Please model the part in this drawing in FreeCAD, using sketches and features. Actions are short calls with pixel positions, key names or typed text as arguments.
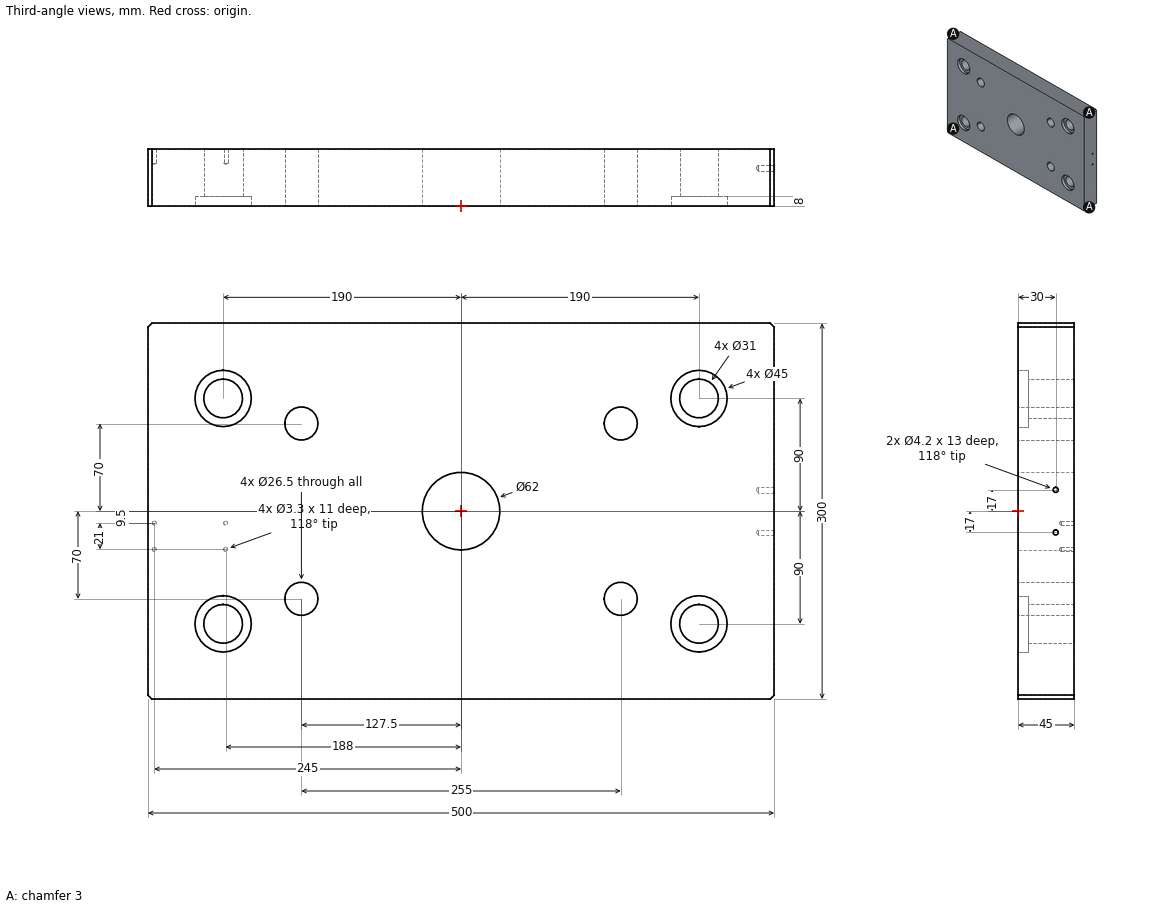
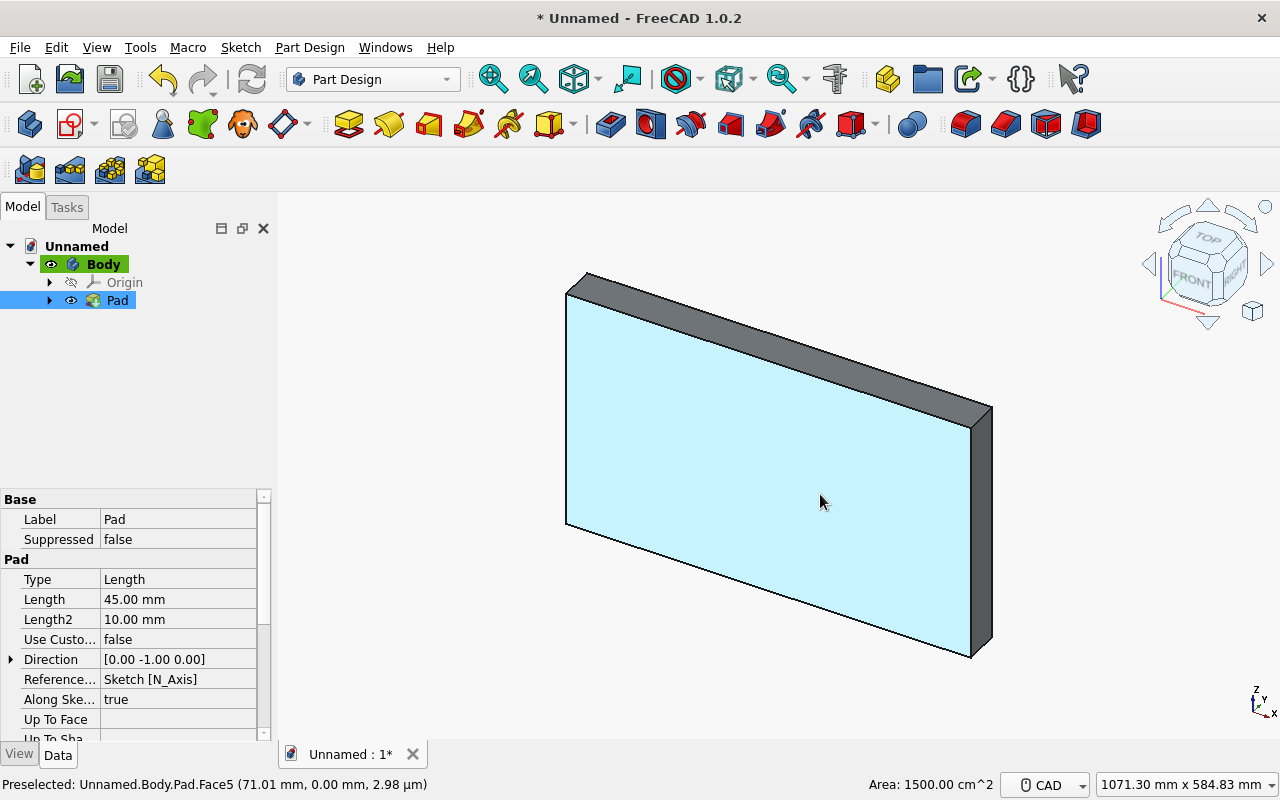
click(70, 124)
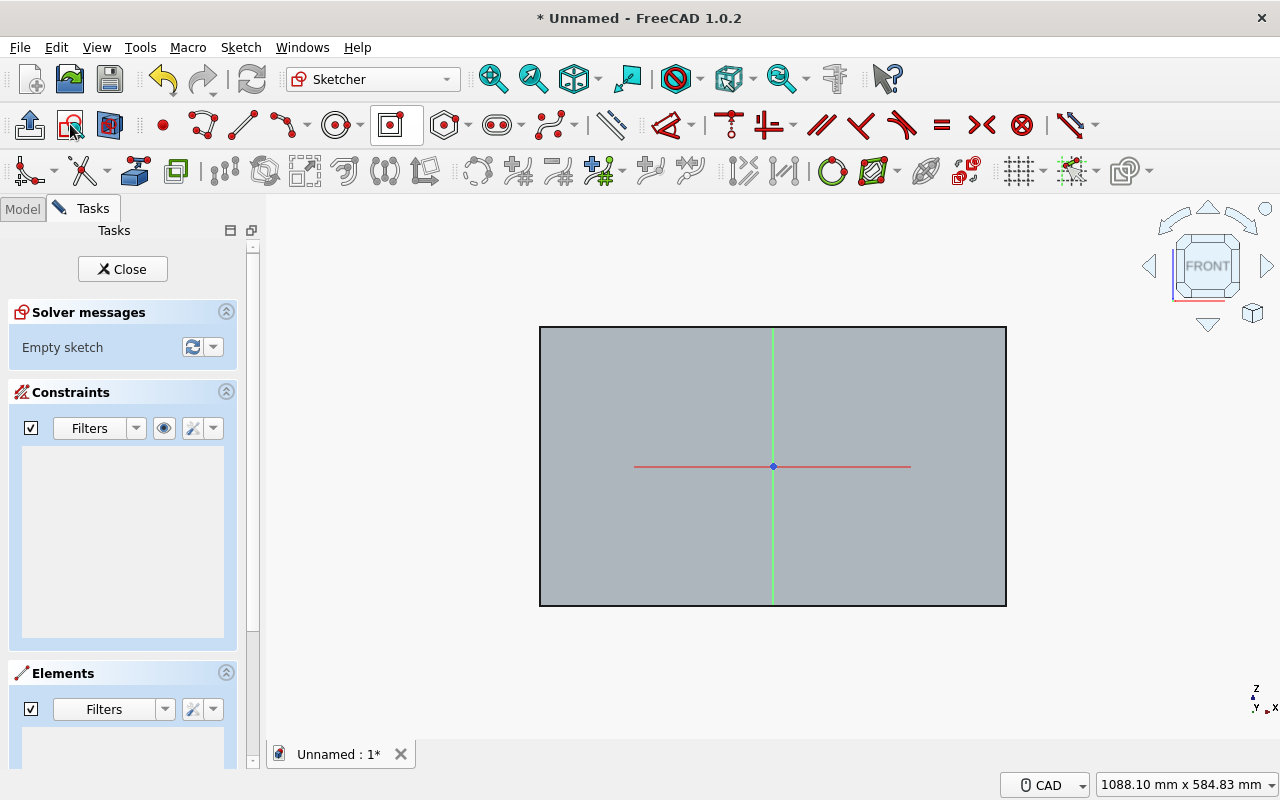
scroll(912, 467, up, 2)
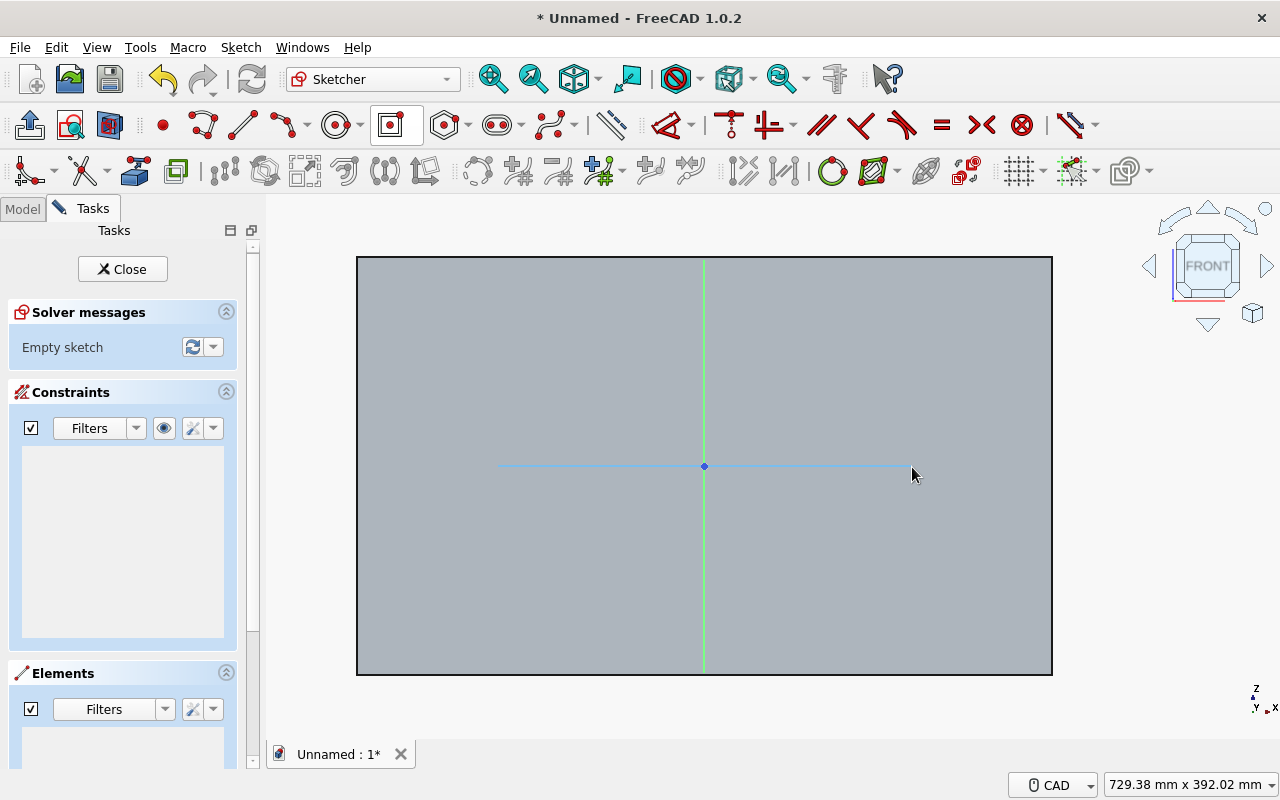
key(g)
key(c)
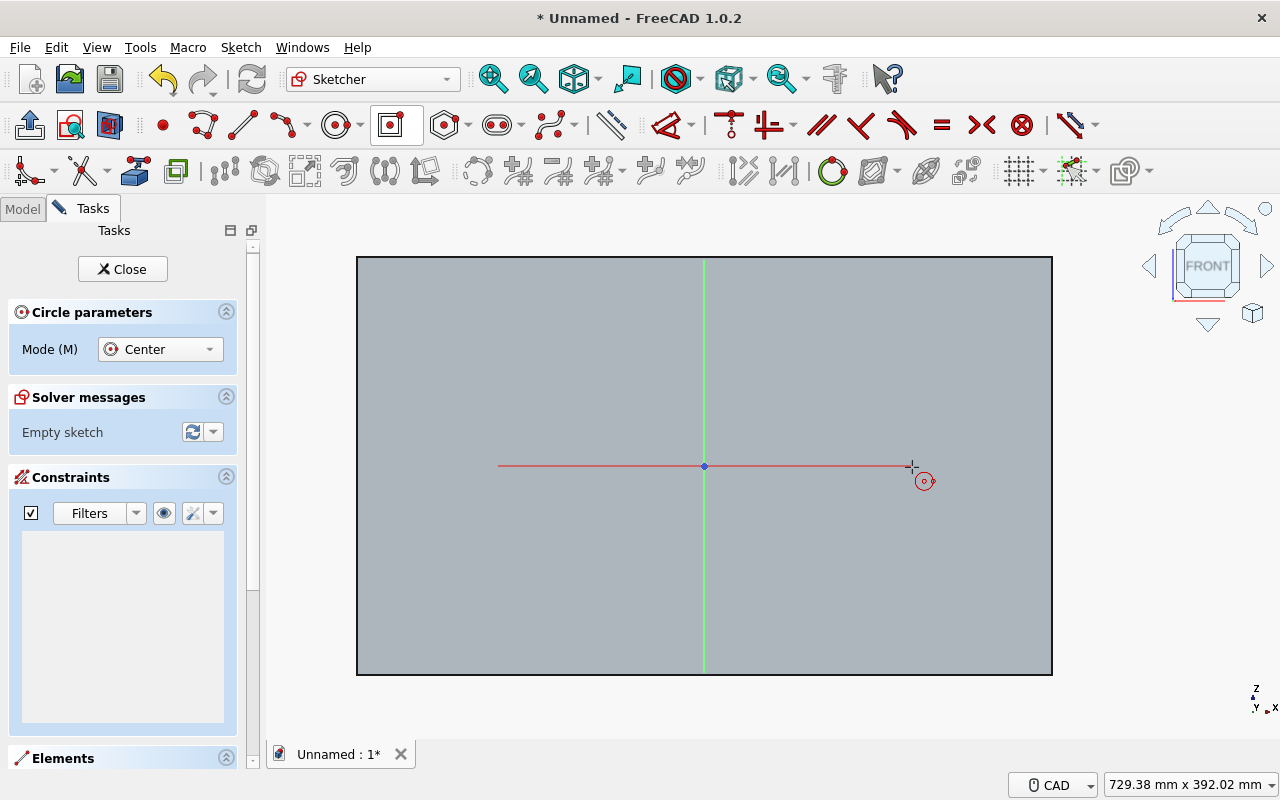
click(968, 341)
click(991, 319)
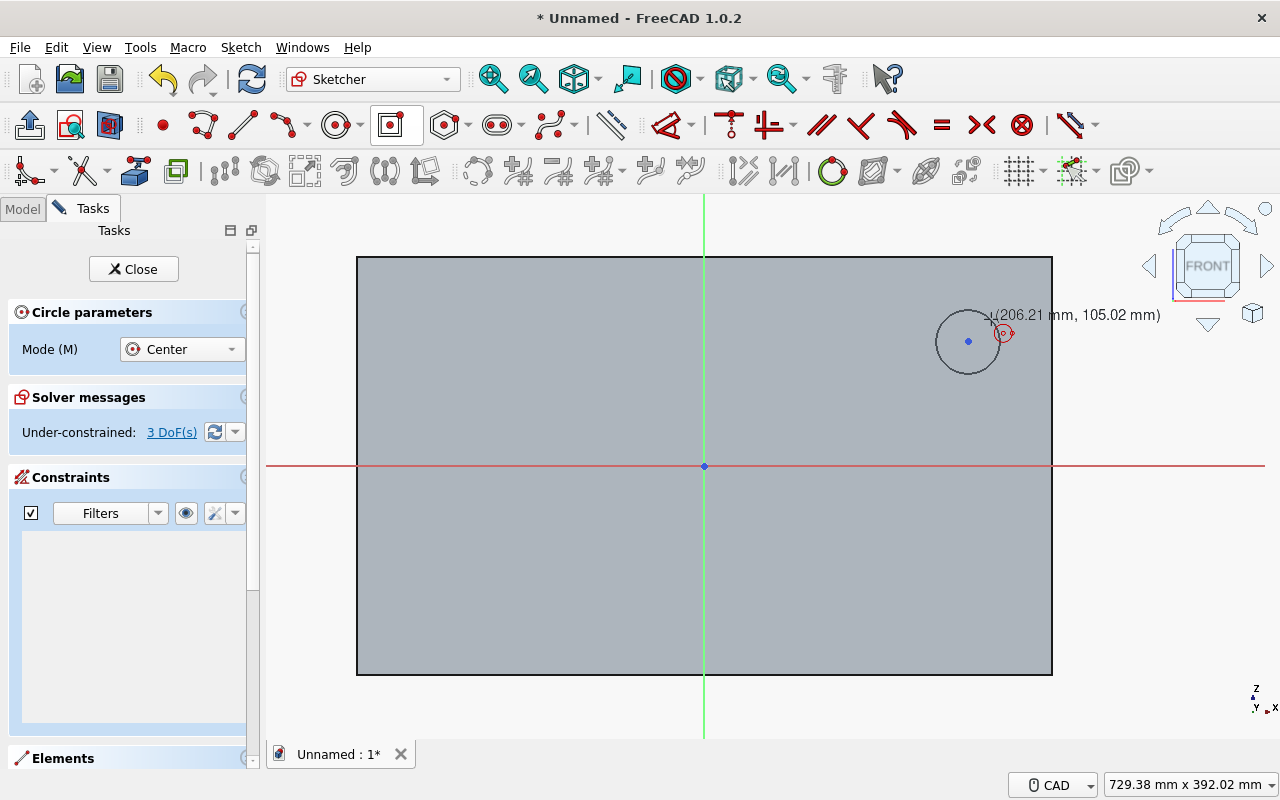
click(440, 341)
click(462, 319)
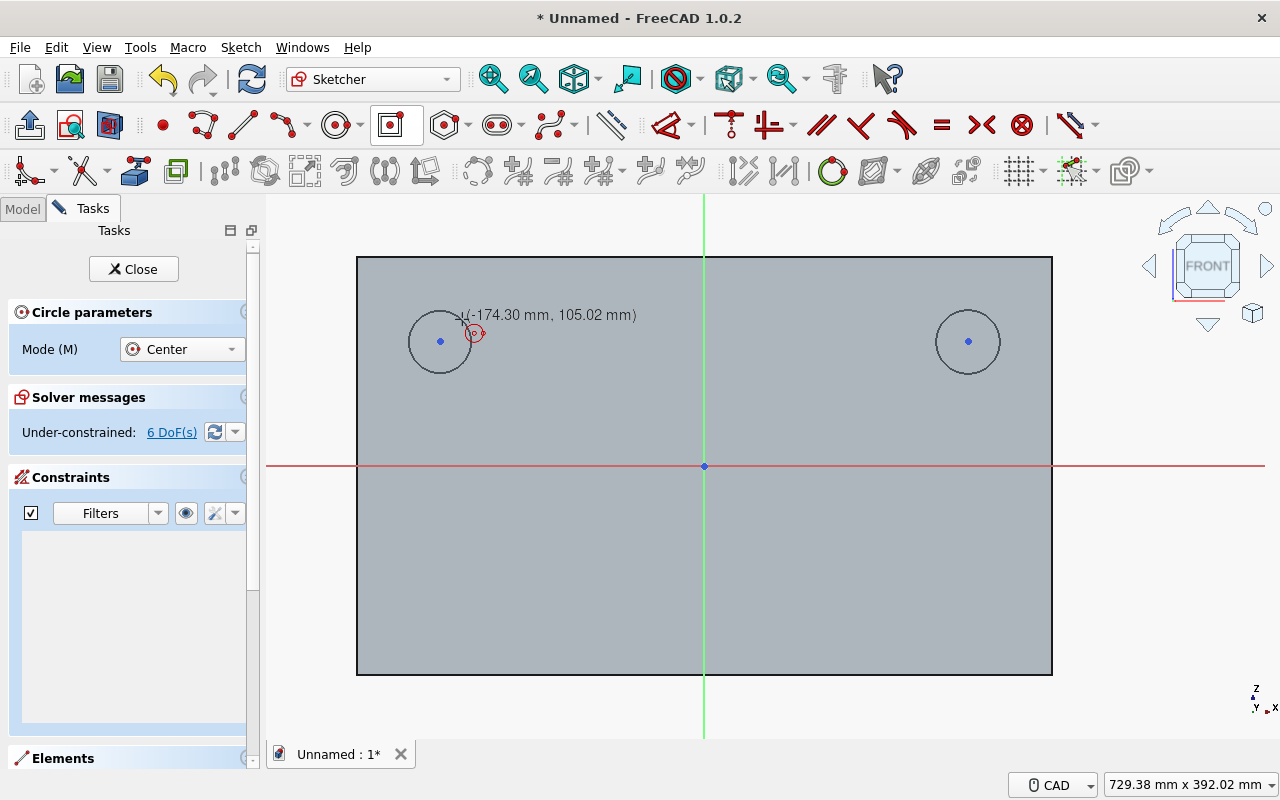
click(968, 591)
click(991, 569)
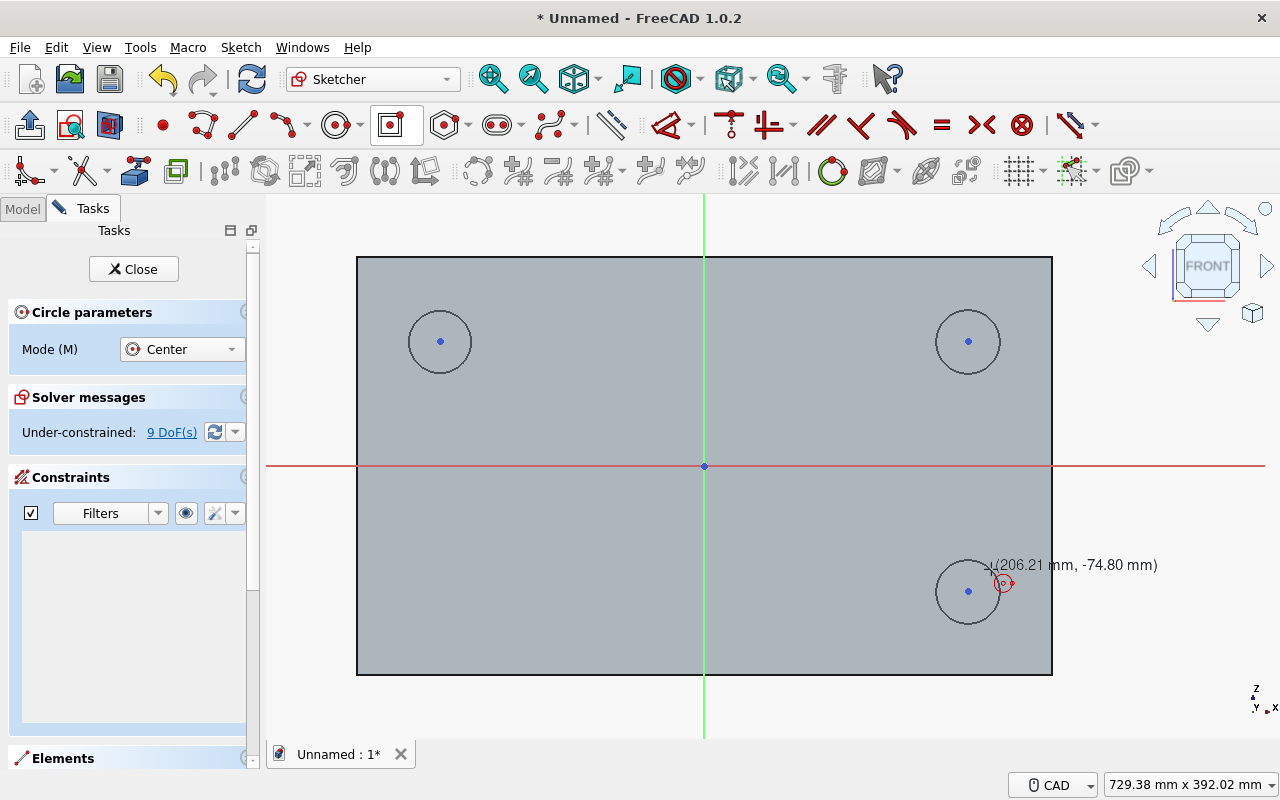
click(440, 591)
click(462, 569)
key(Escape)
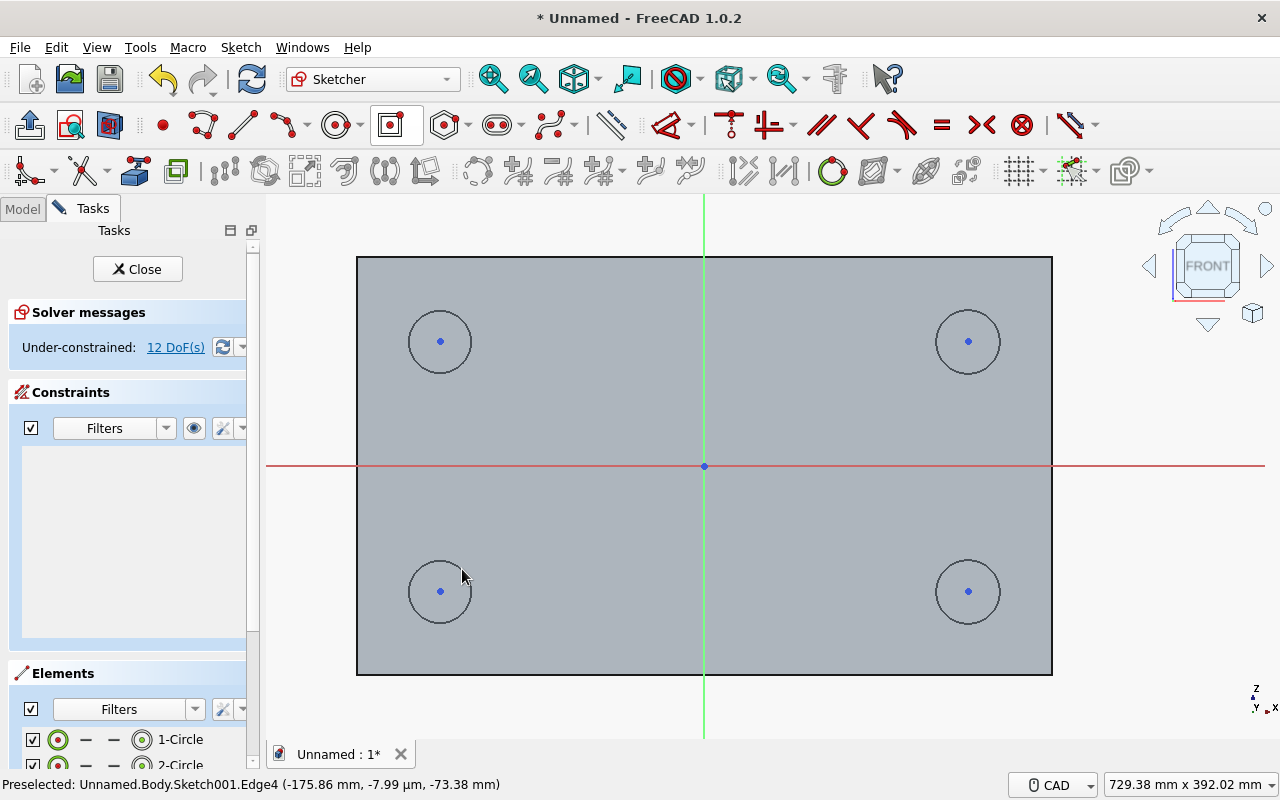
click(990, 319)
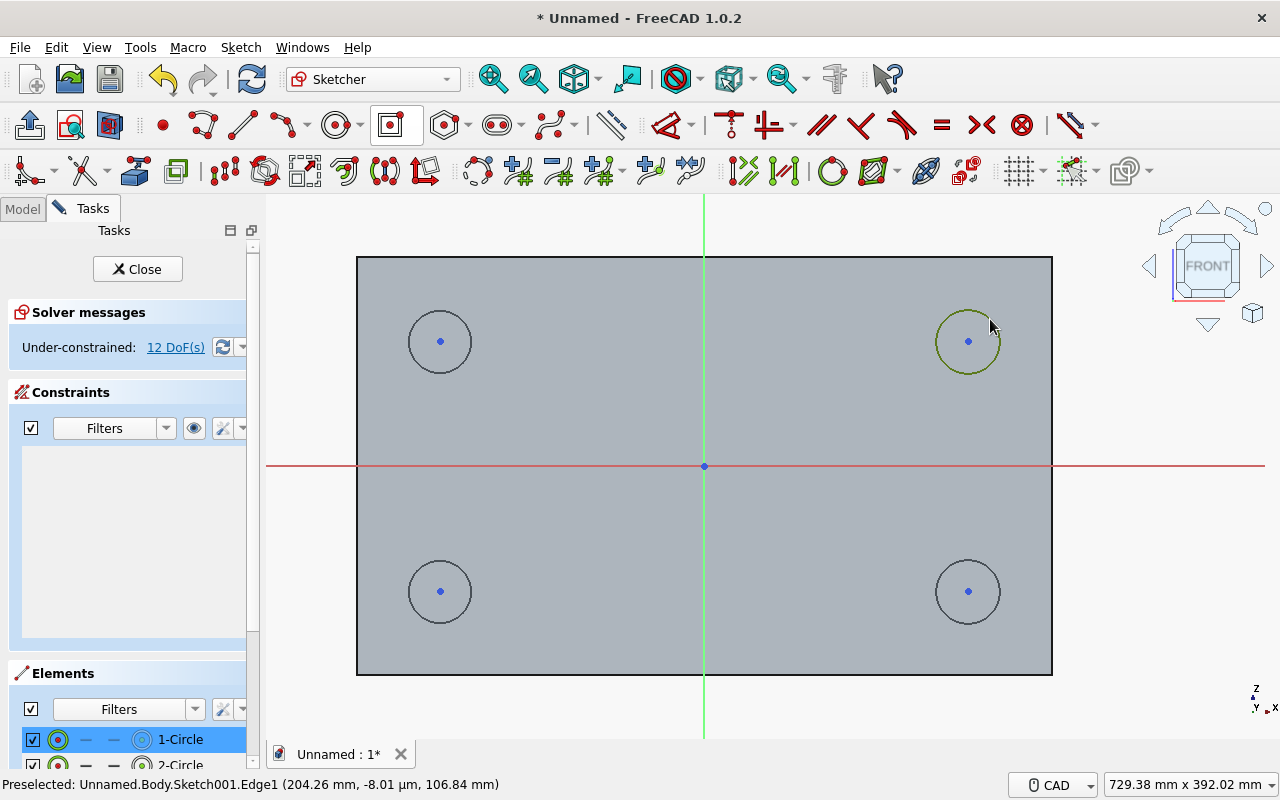
click(462, 320)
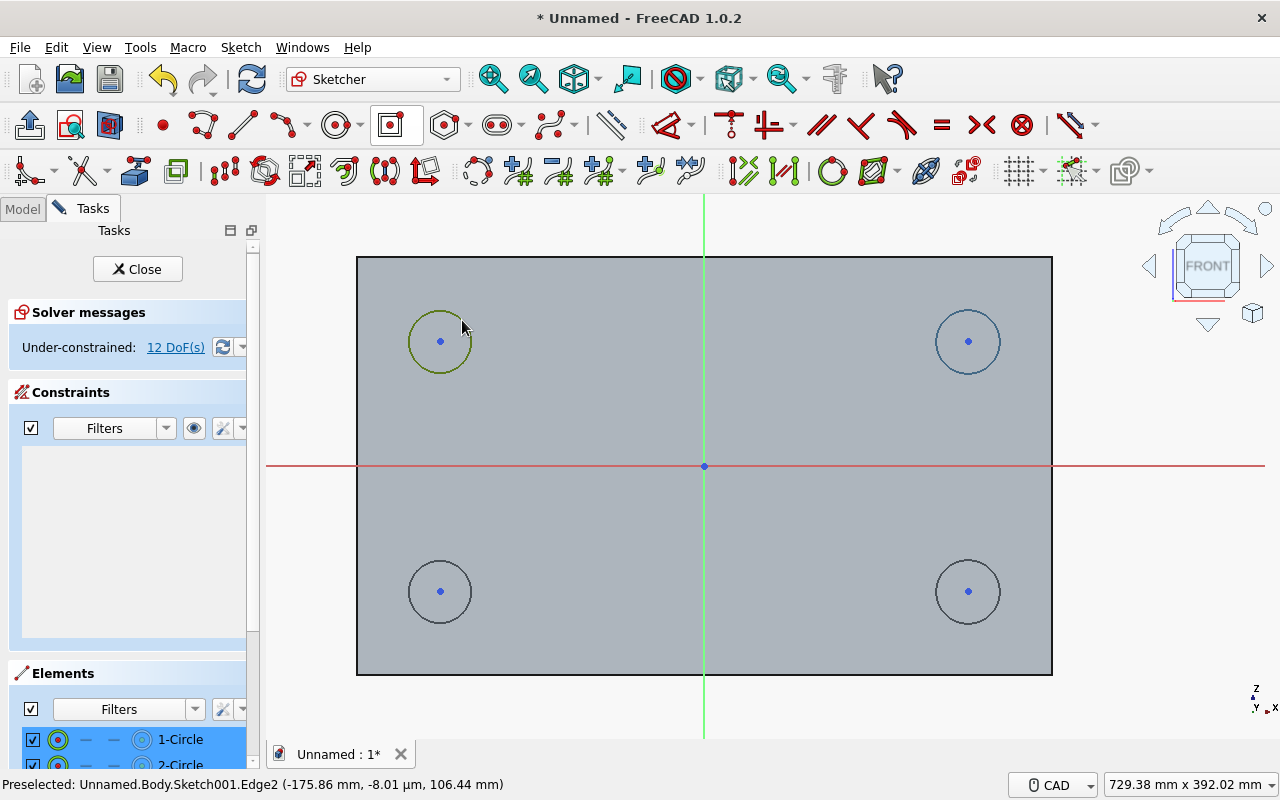
click(990, 569)